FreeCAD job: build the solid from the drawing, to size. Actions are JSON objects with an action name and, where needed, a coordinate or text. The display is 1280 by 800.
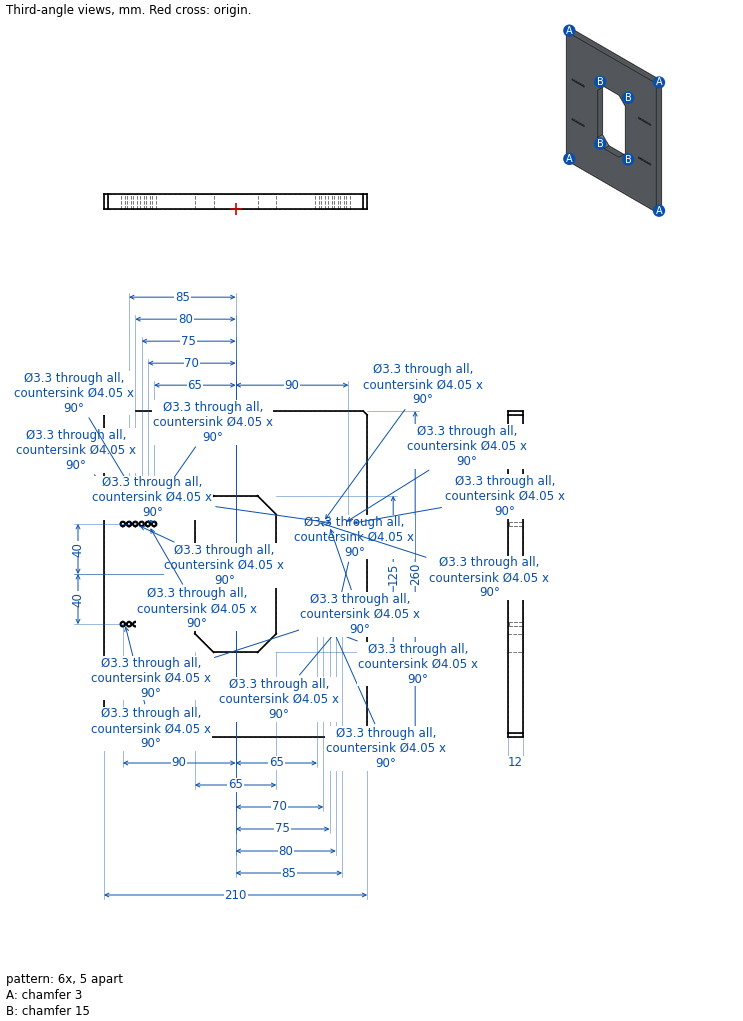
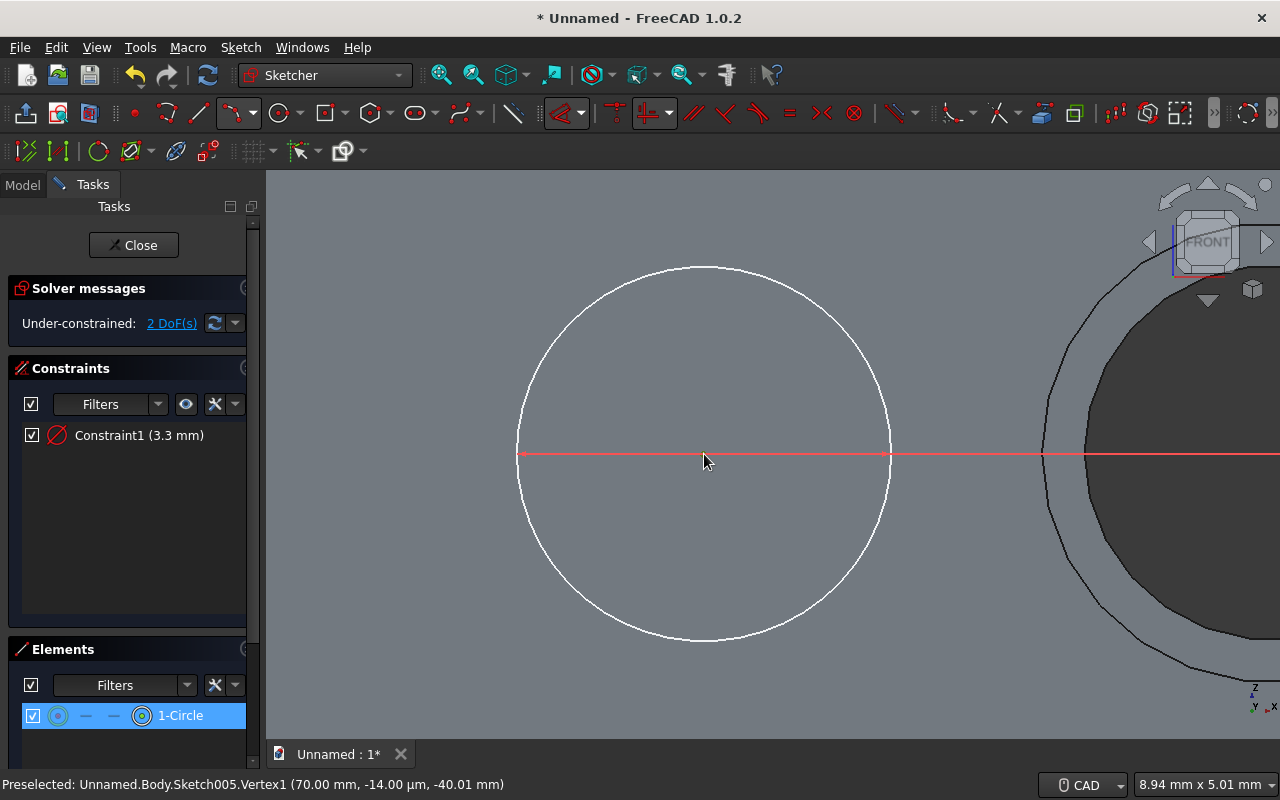
{"action": "left_click", "coordinate": [584, 114]}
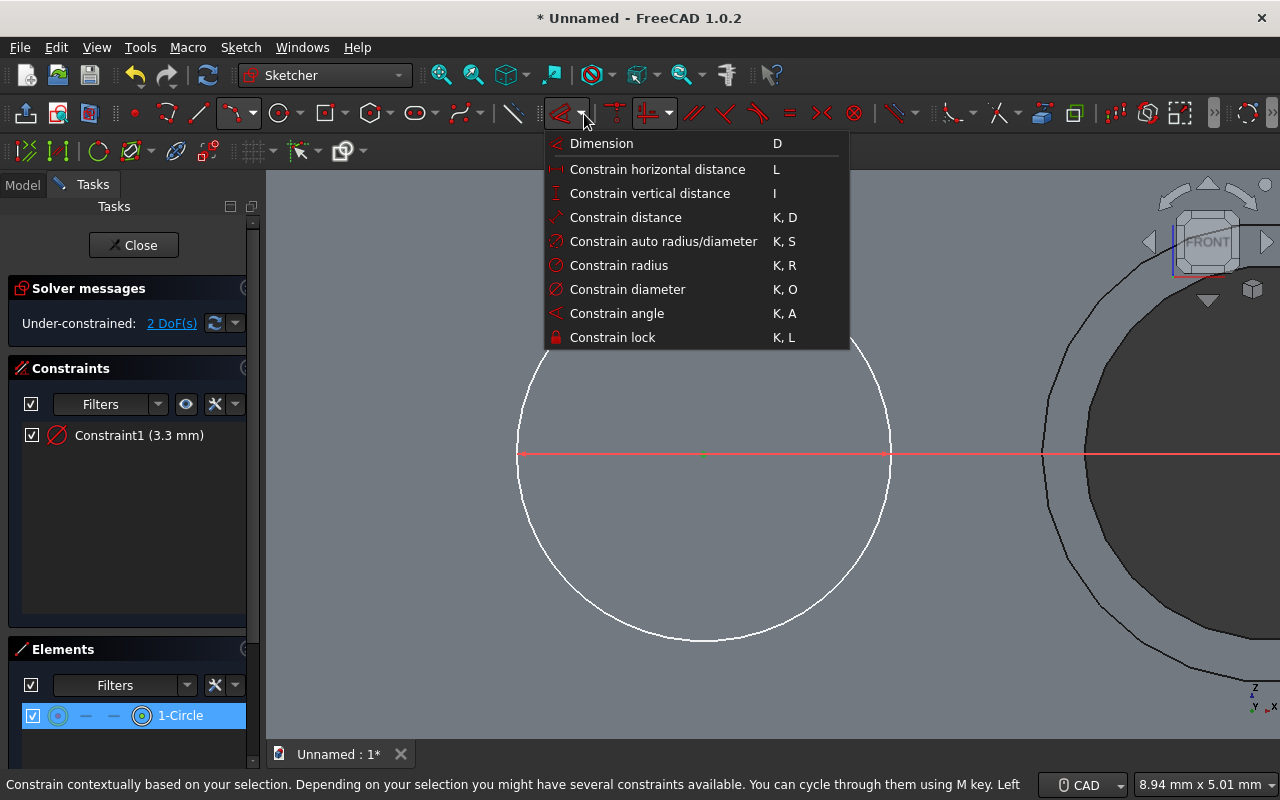
{"action": "left_click", "coordinate": [697, 169]}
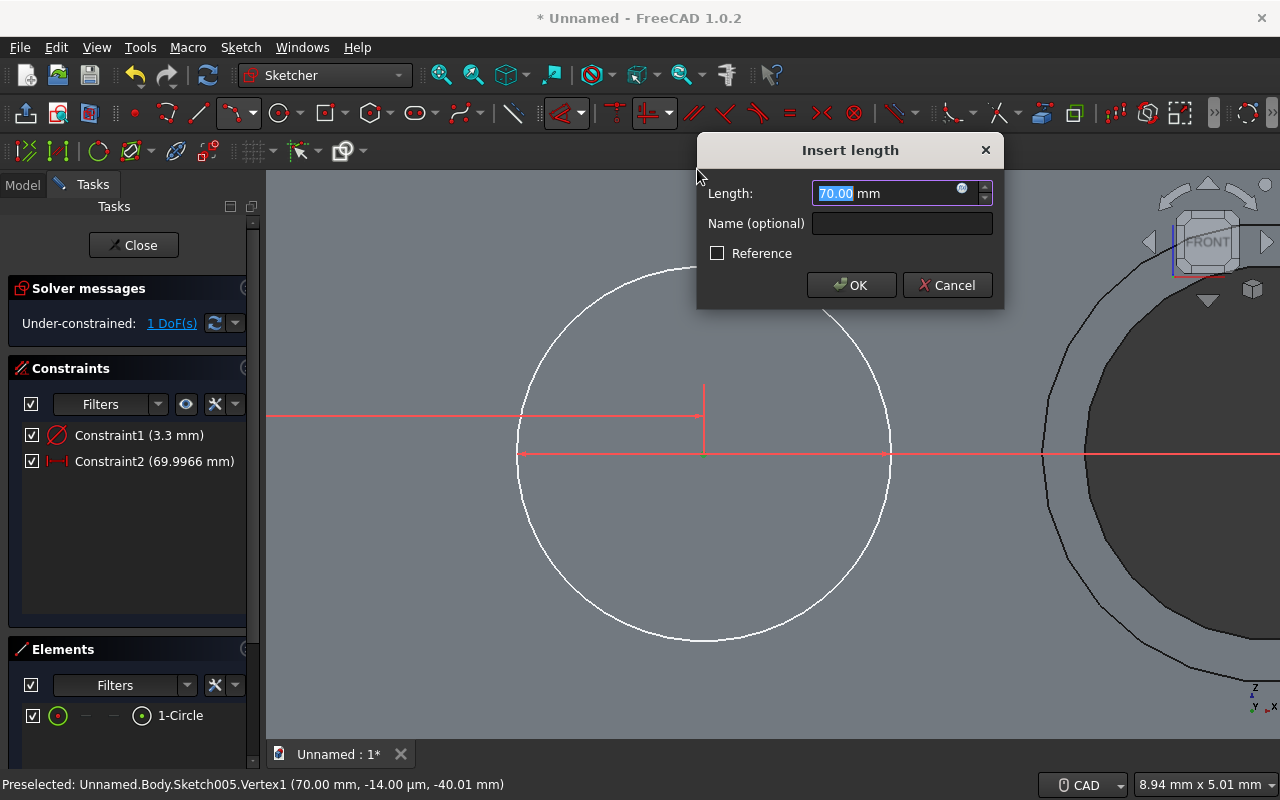
{"action": "type", "text": "70"}
{"action": "key", "text": "Return"}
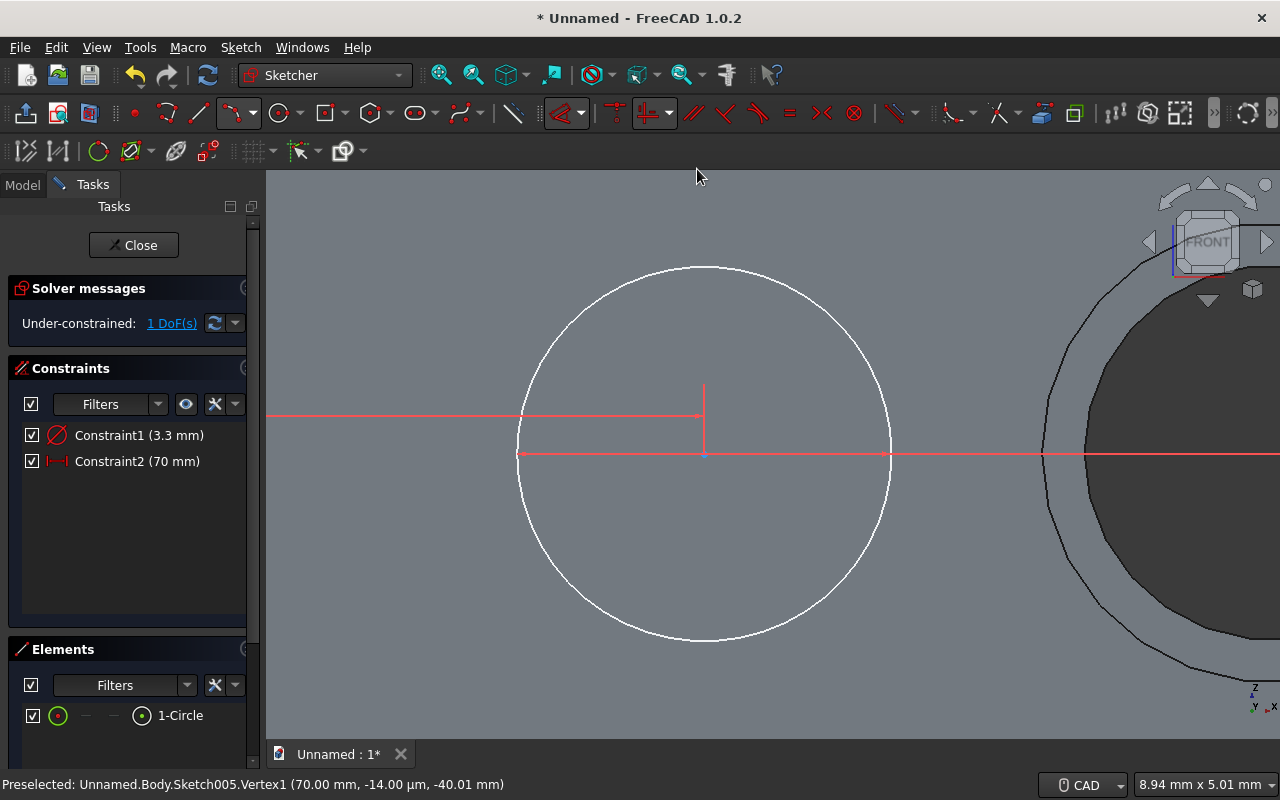
{"action": "left_click", "coordinate": [704, 454]}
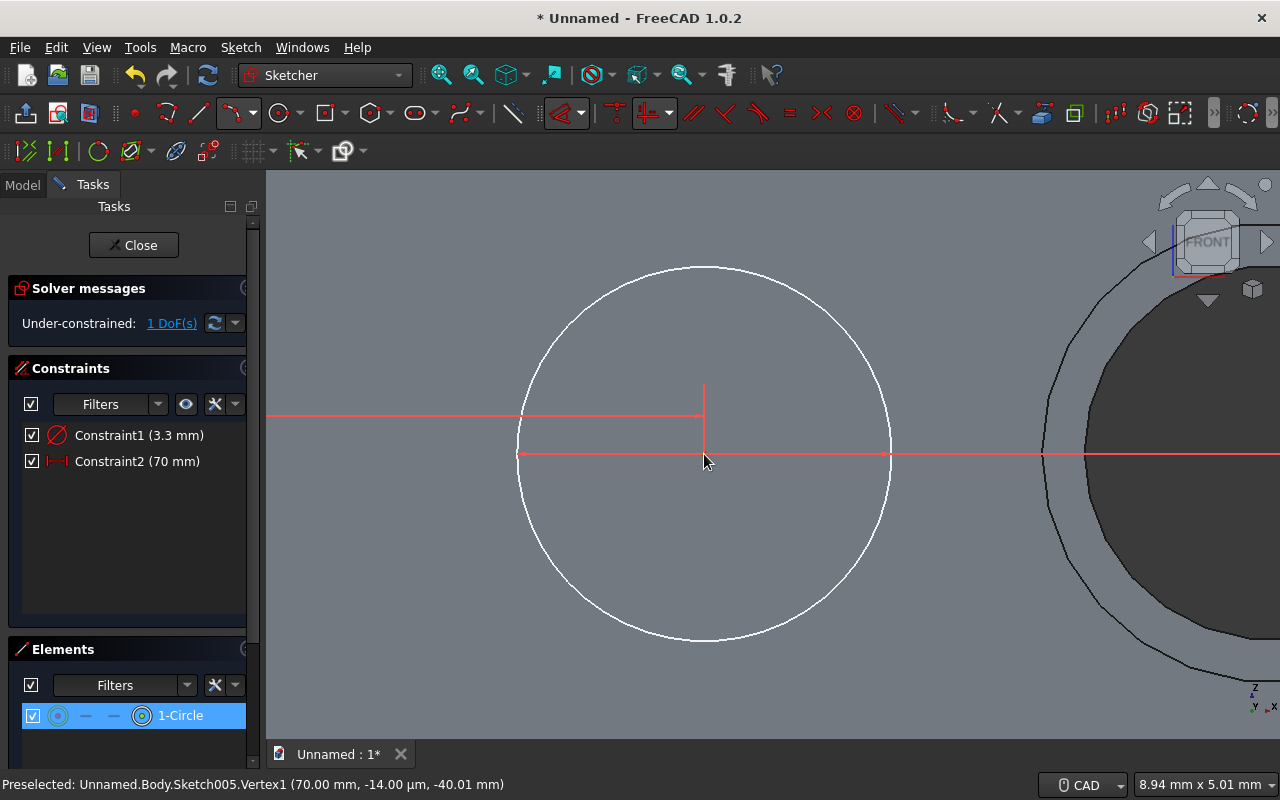
{"action": "key", "text": "i"}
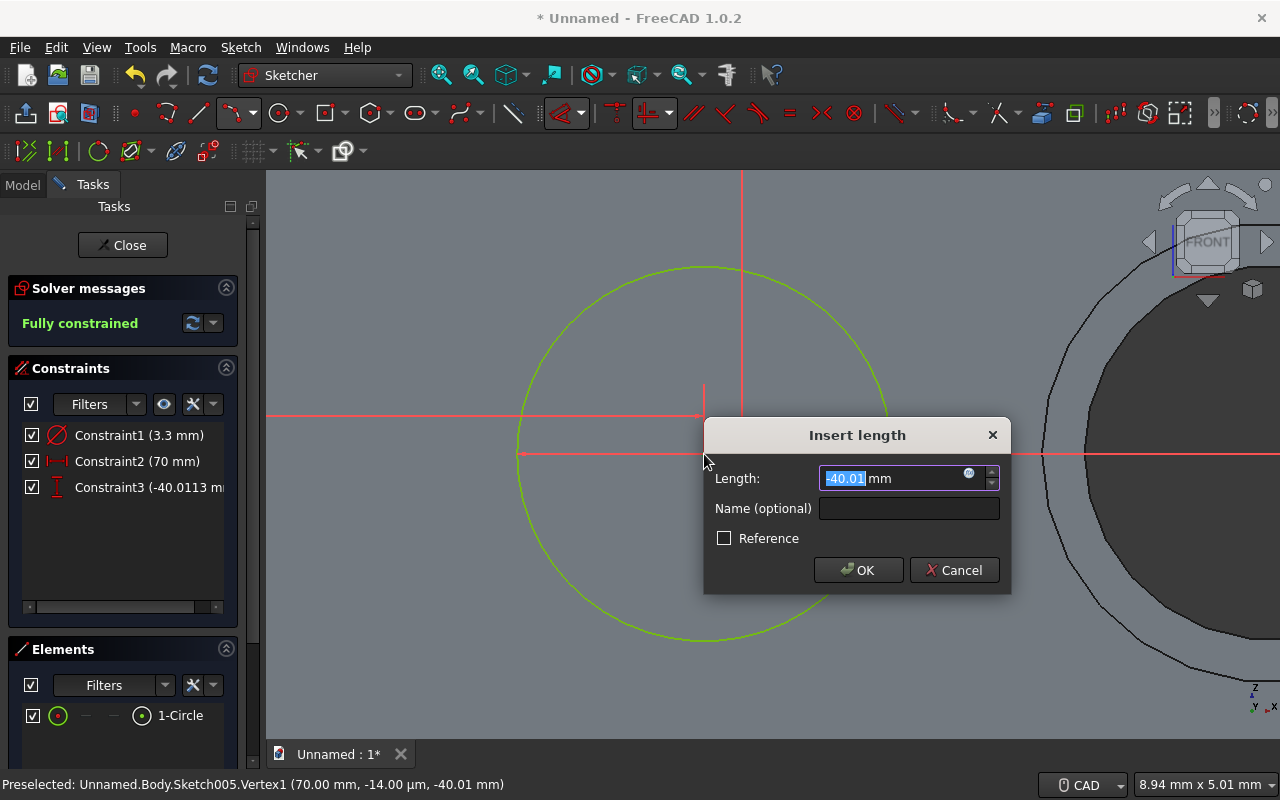
{"action": "type", "text": "-40"}
{"action": "key", "text": "Return"}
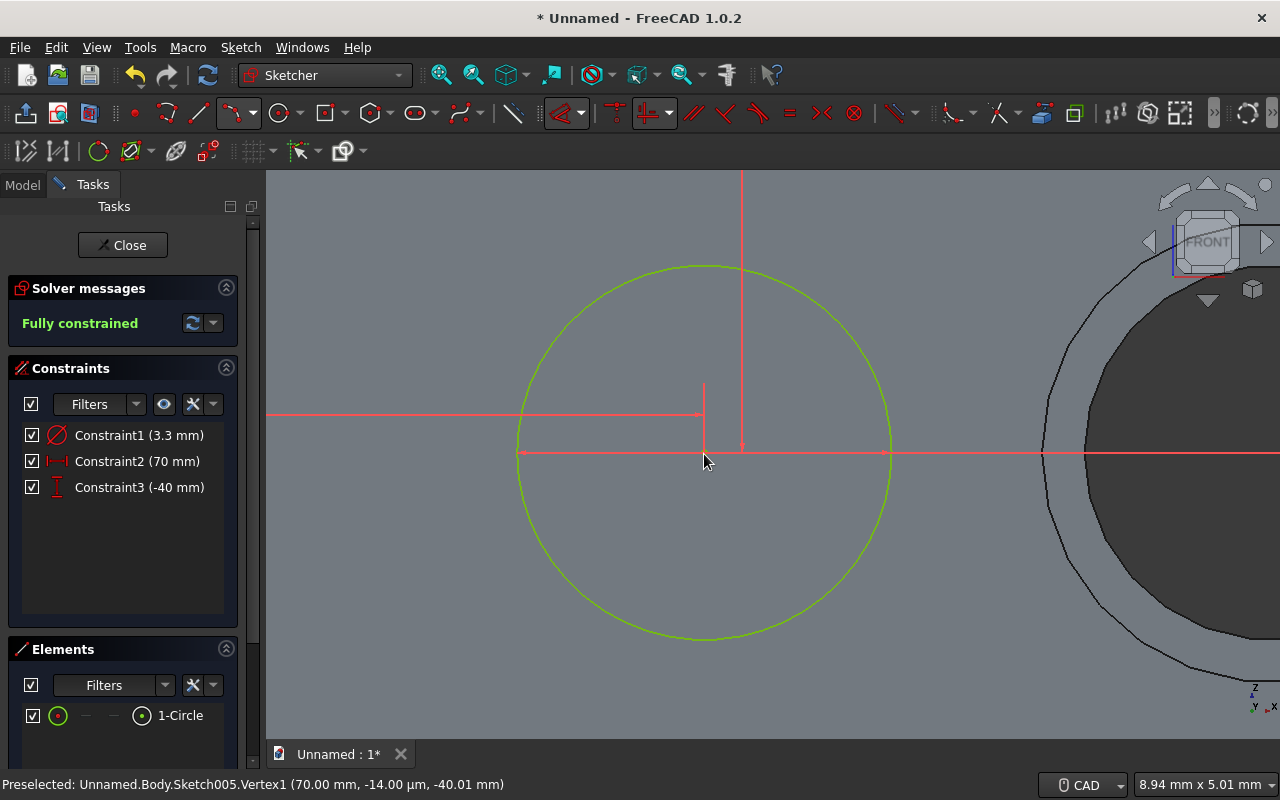
{"action": "left_click", "coordinate": [123, 245]}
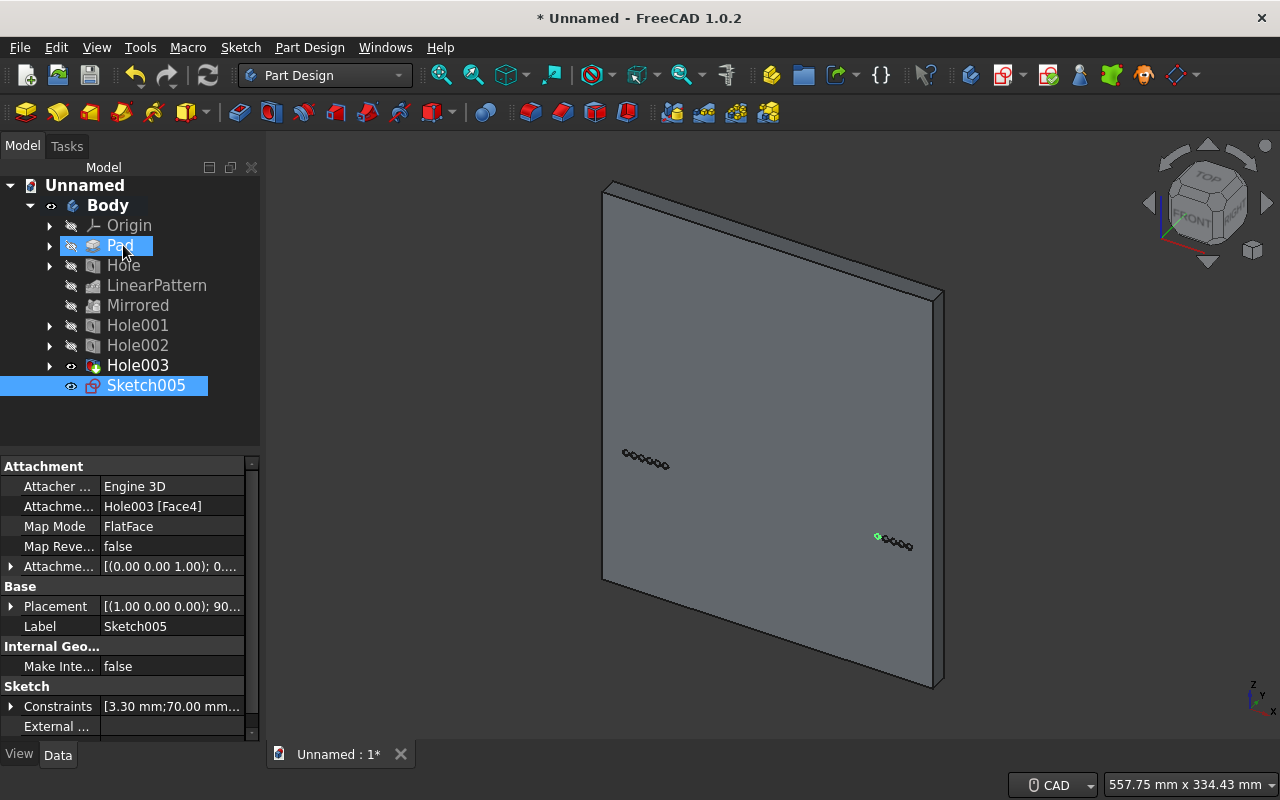
{"action": "left_click", "coordinate": [272, 112]}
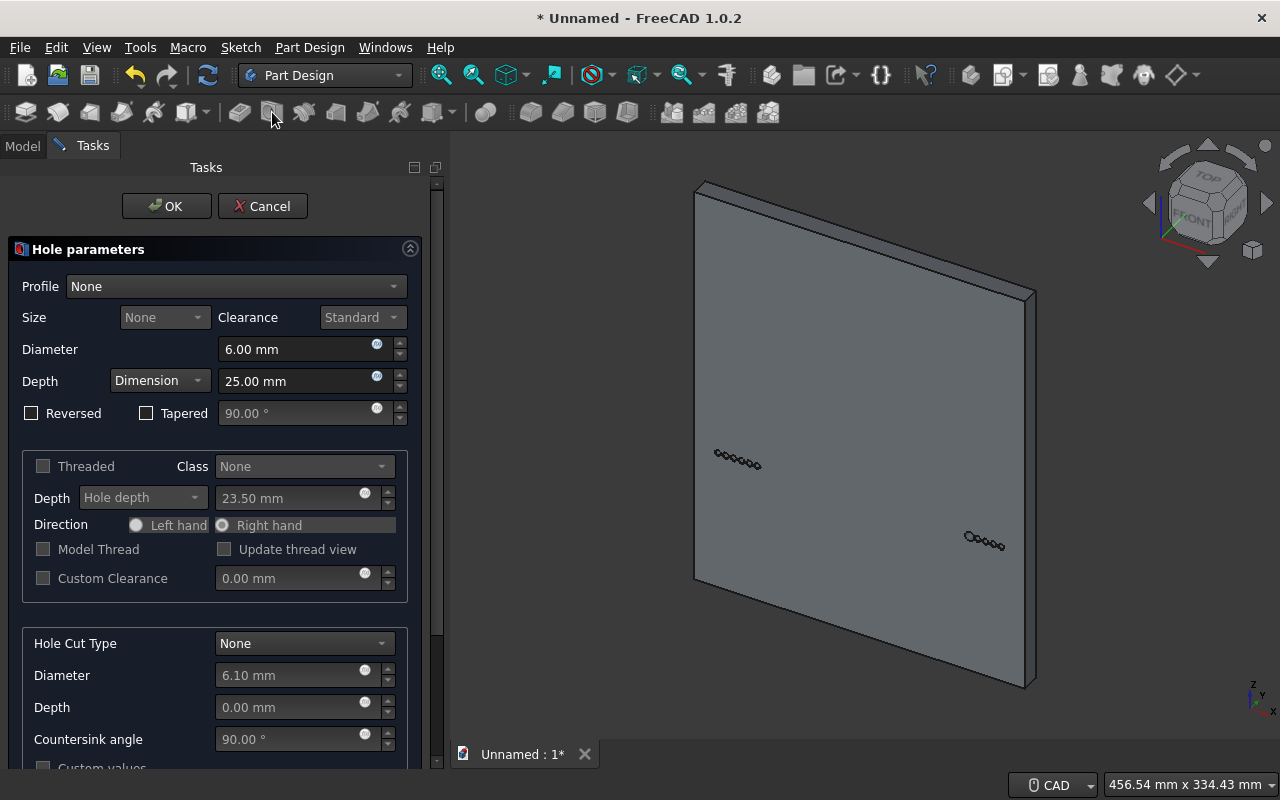
{"action": "triple_click", "coordinate": [305, 349]}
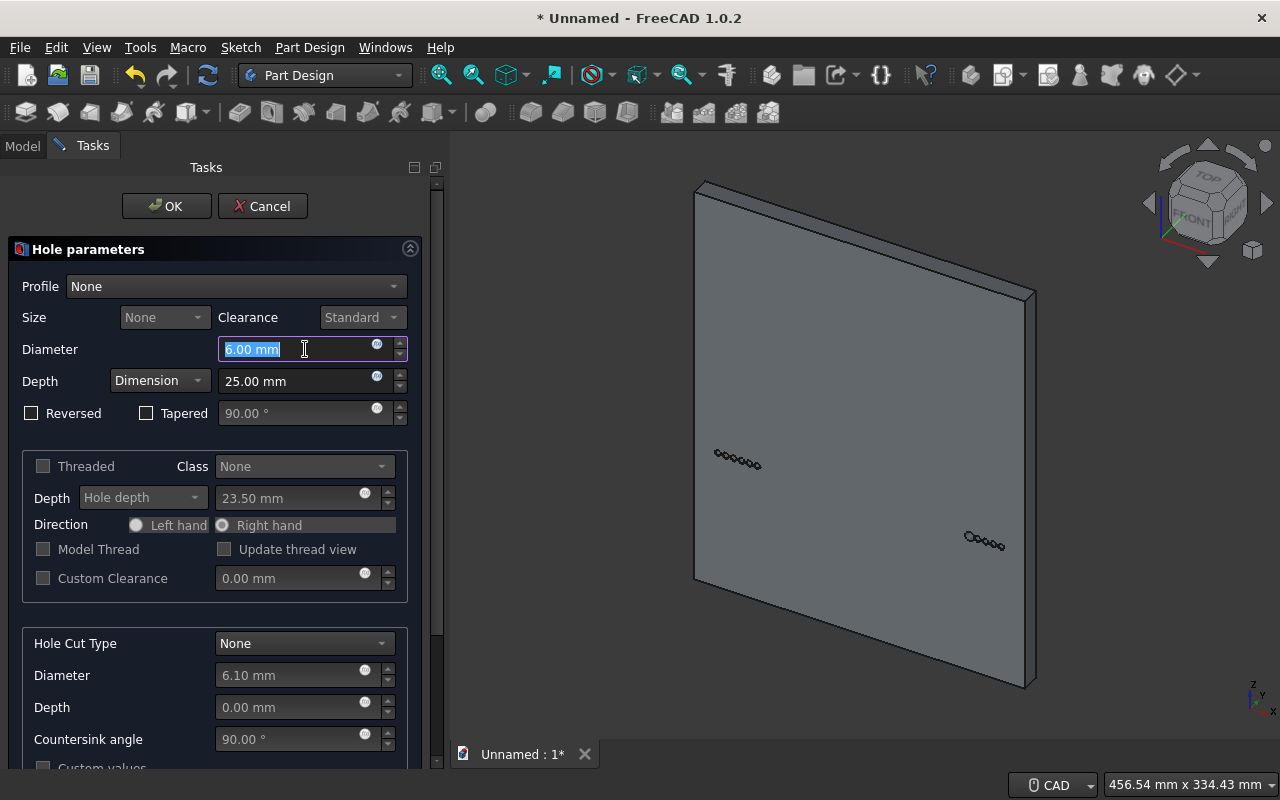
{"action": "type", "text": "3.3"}
{"action": "key", "text": "Tab"}